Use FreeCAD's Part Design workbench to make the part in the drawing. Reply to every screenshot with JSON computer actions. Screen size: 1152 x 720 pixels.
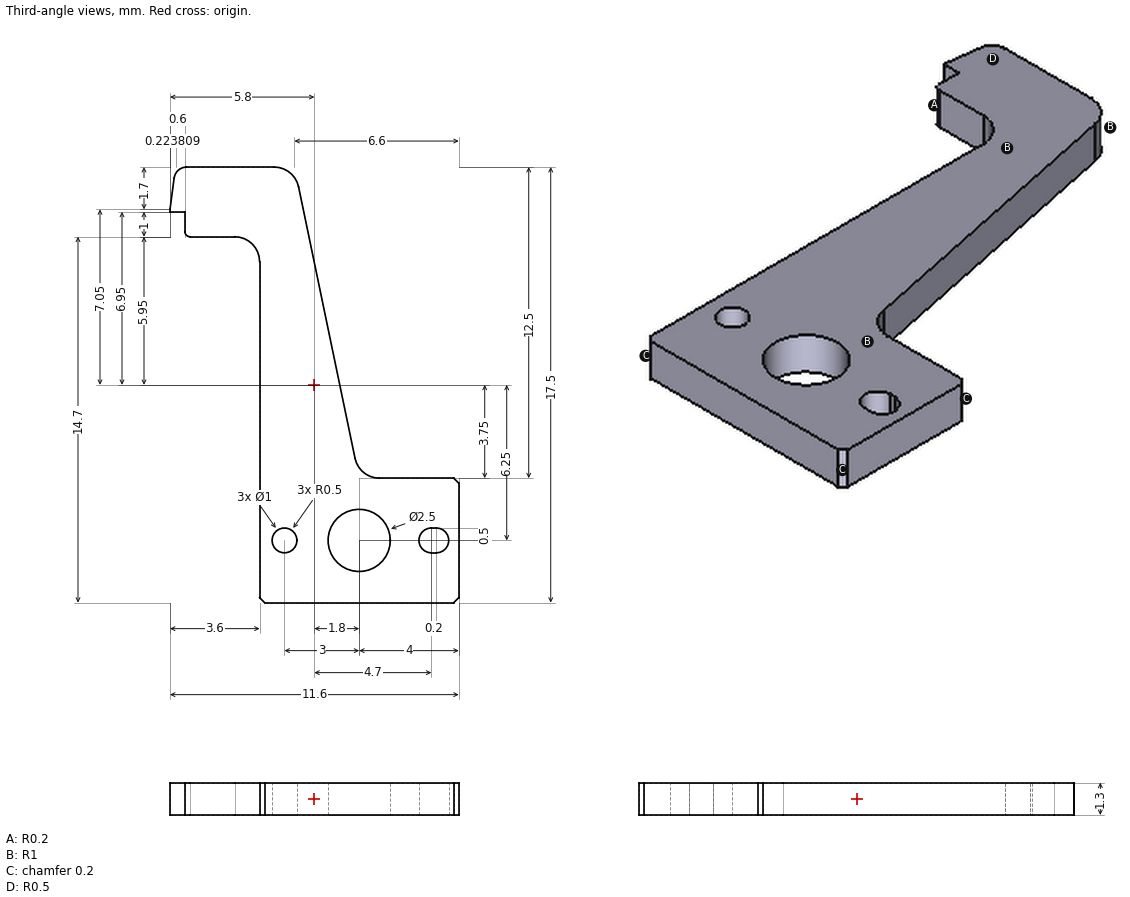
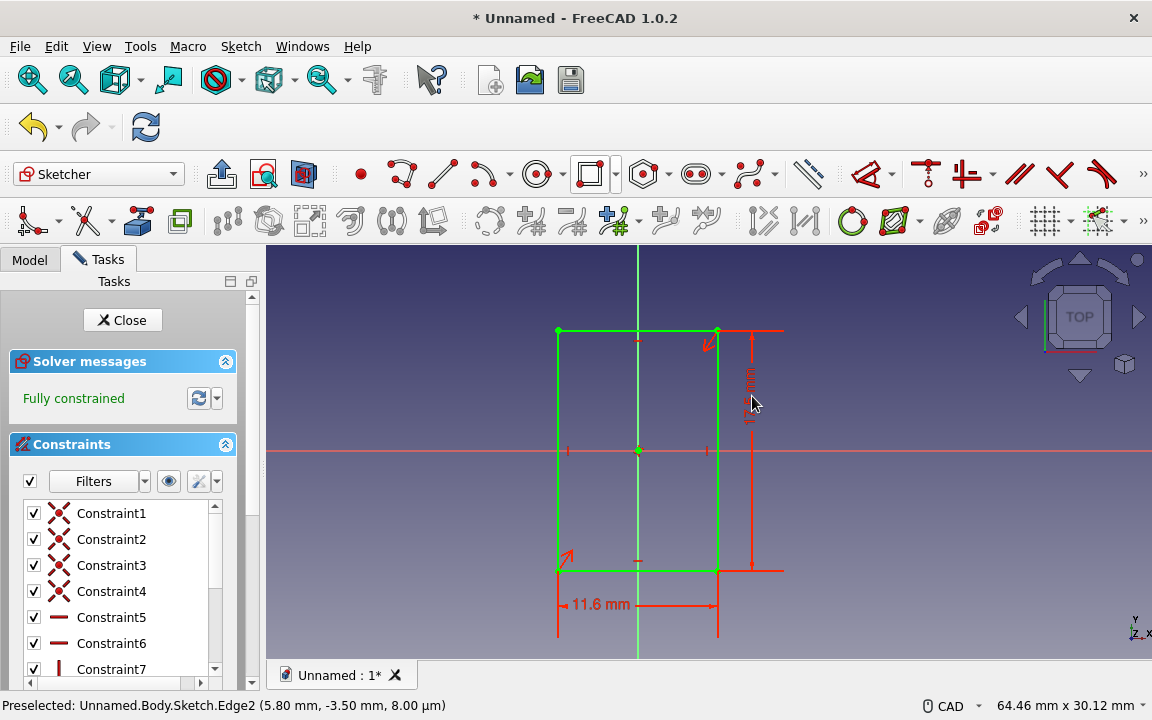
{"action": "left_click", "coordinate": [123, 320]}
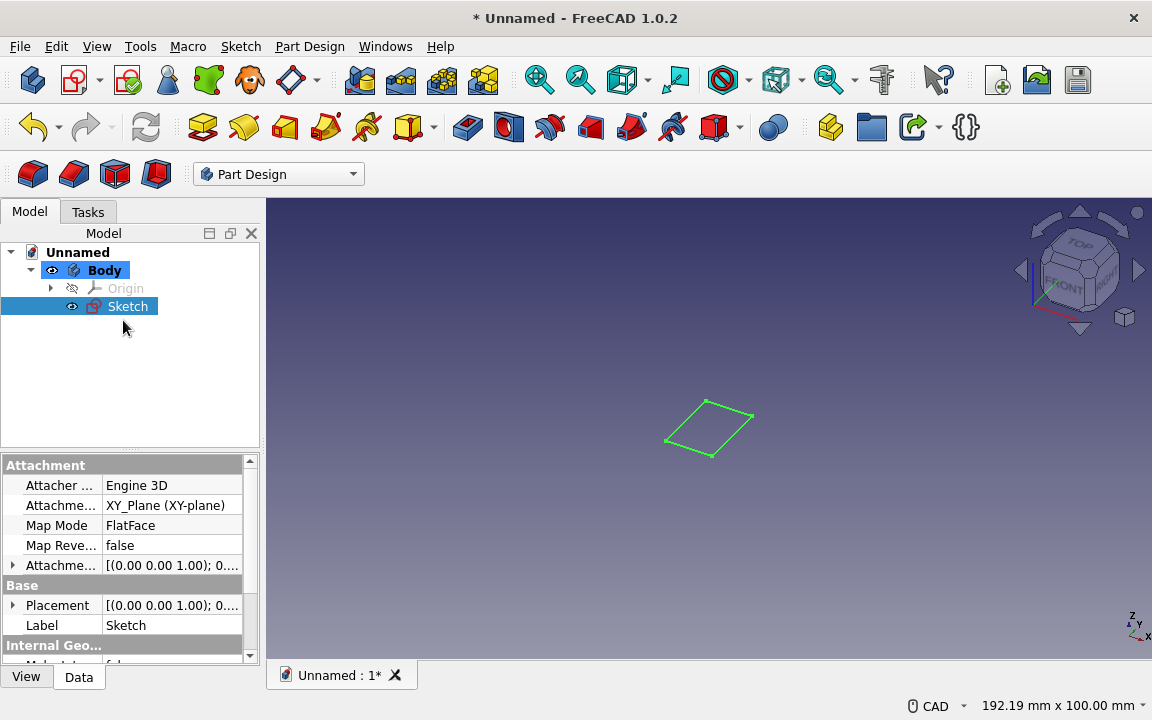
{"action": "left_click", "coordinate": [203, 128]}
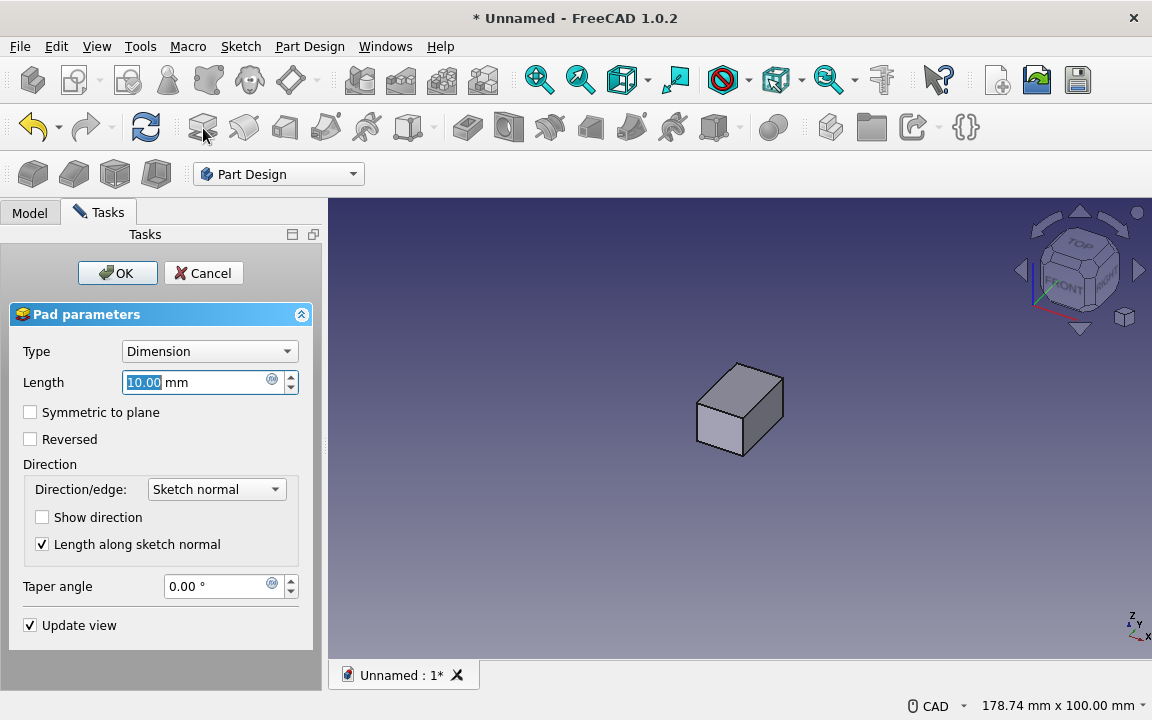
{"action": "type", "text": "1.3"}
{"action": "key", "text": "Tab"}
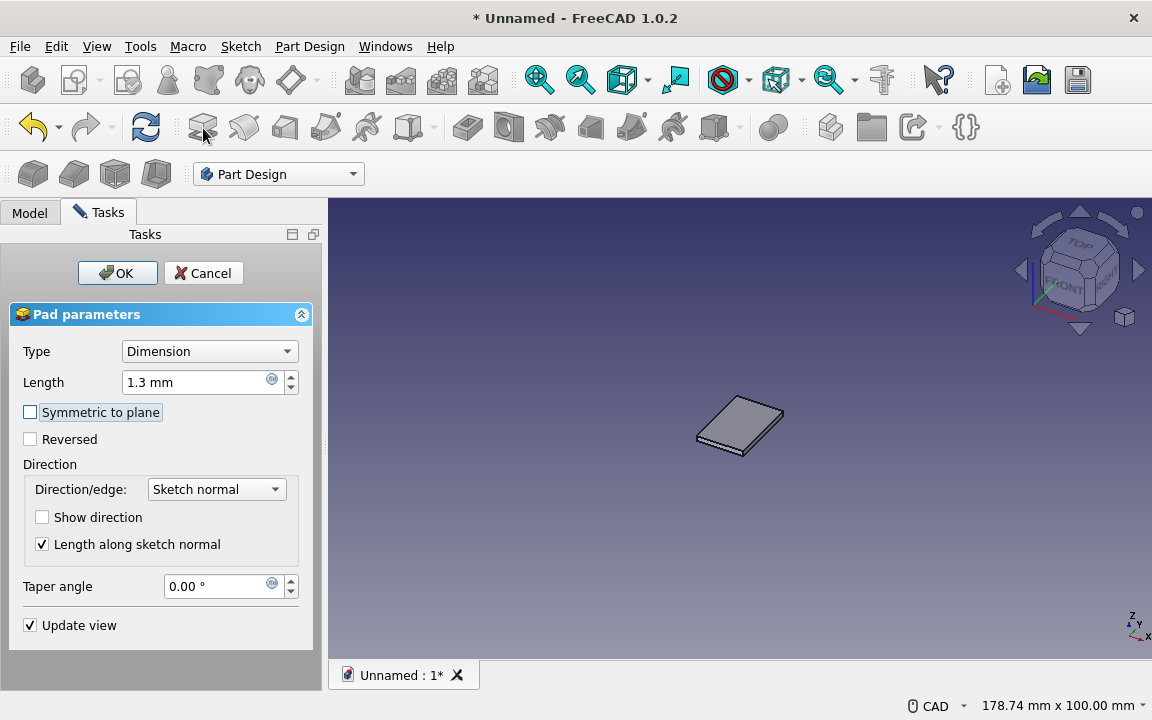
{"action": "left_click", "coordinate": [31, 412]}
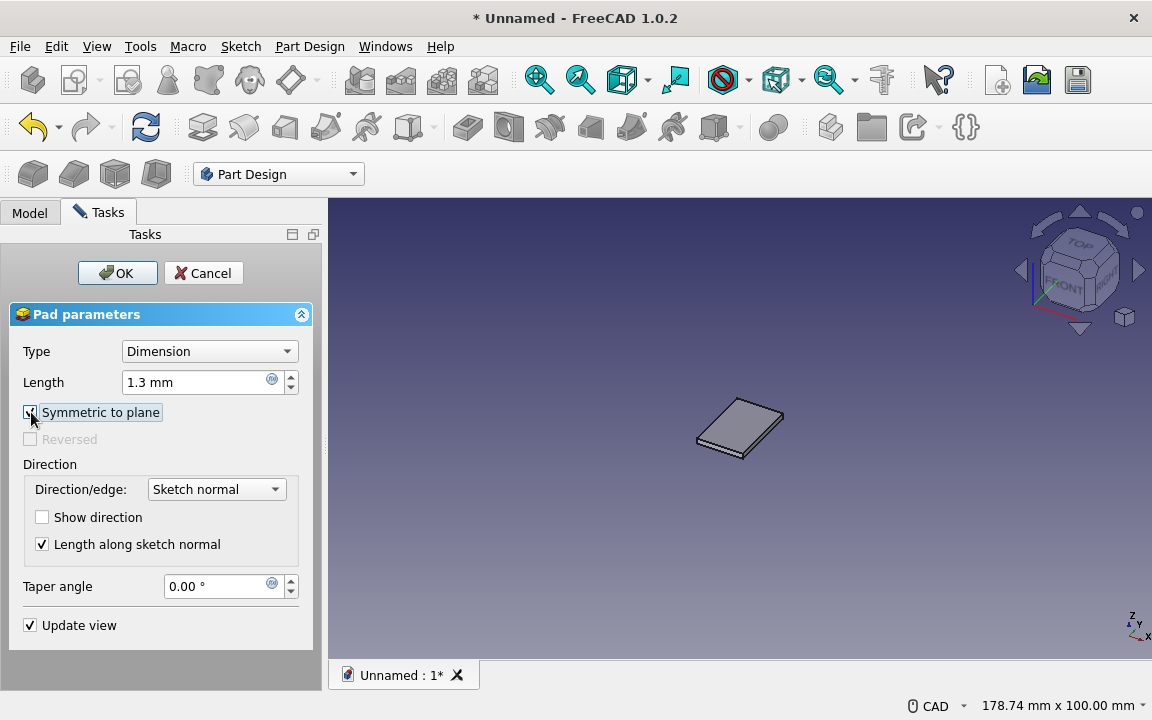
{"action": "left_click", "coordinate": [118, 273]}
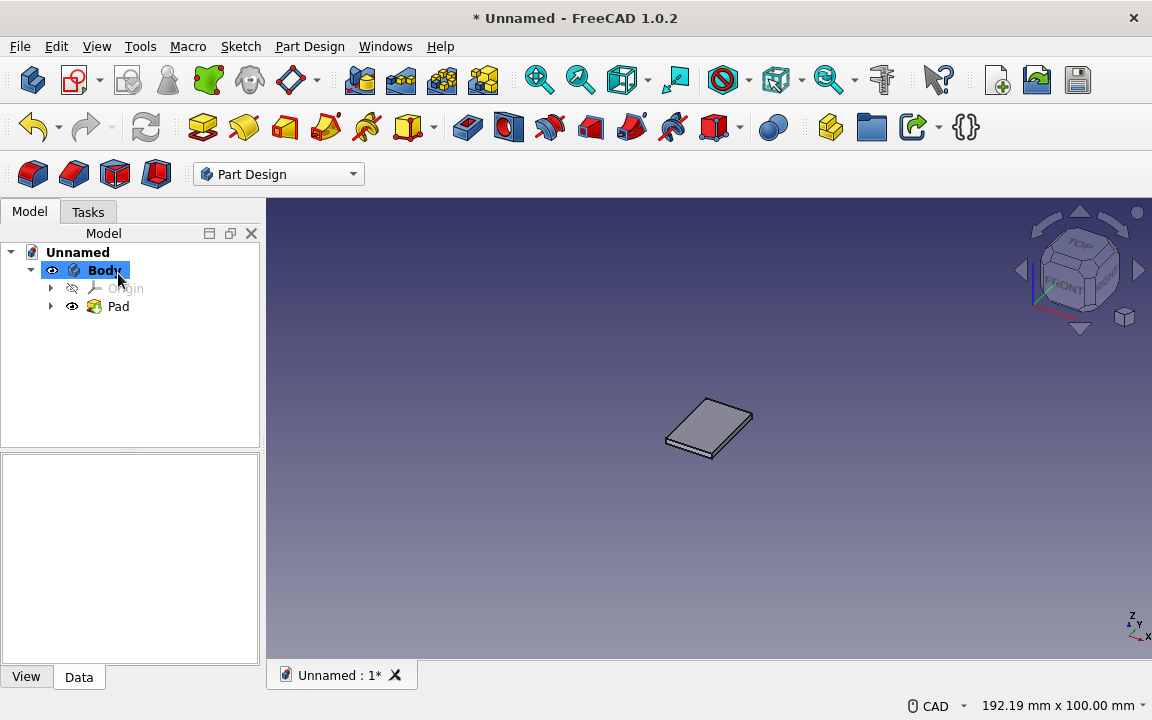
{"action": "key", "text": "v f"}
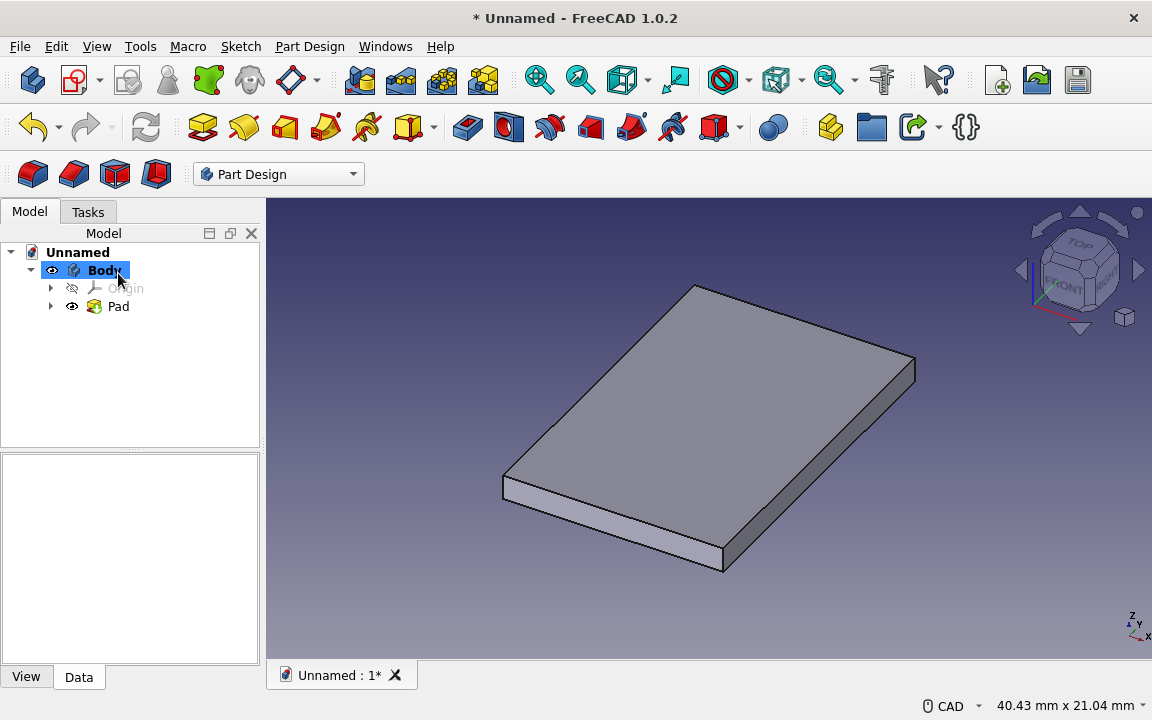
{"action": "left_click", "coordinate": [736, 389]}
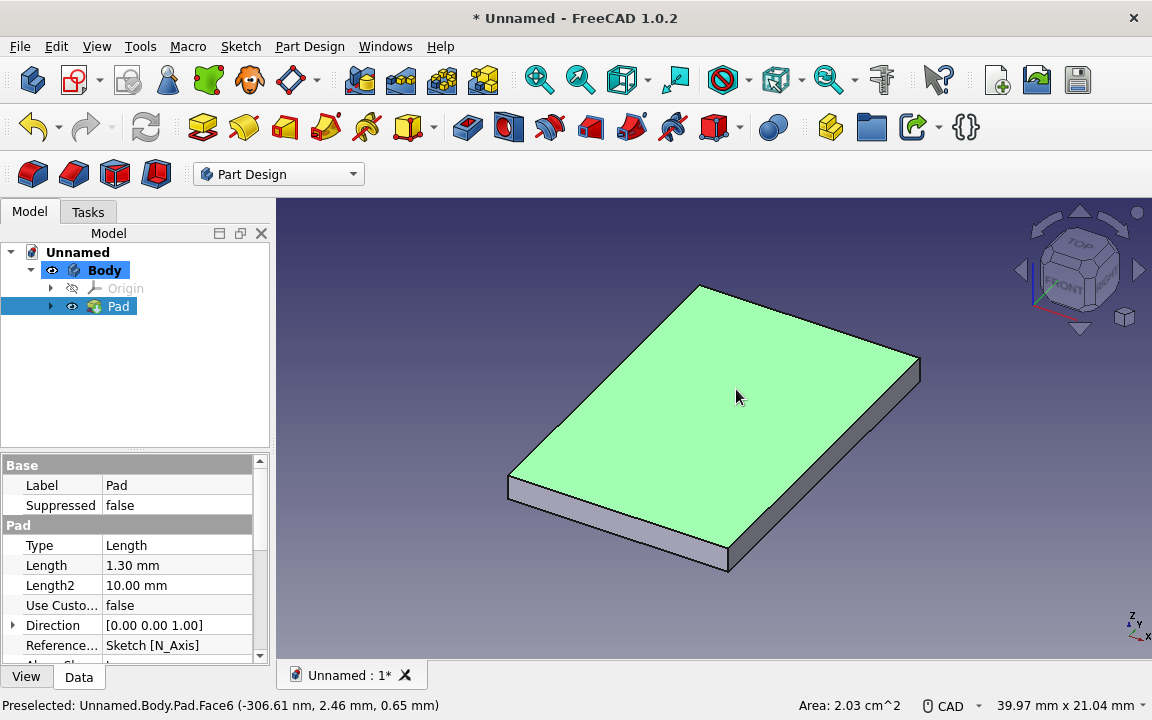
{"action": "left_click", "coordinate": [74, 80]}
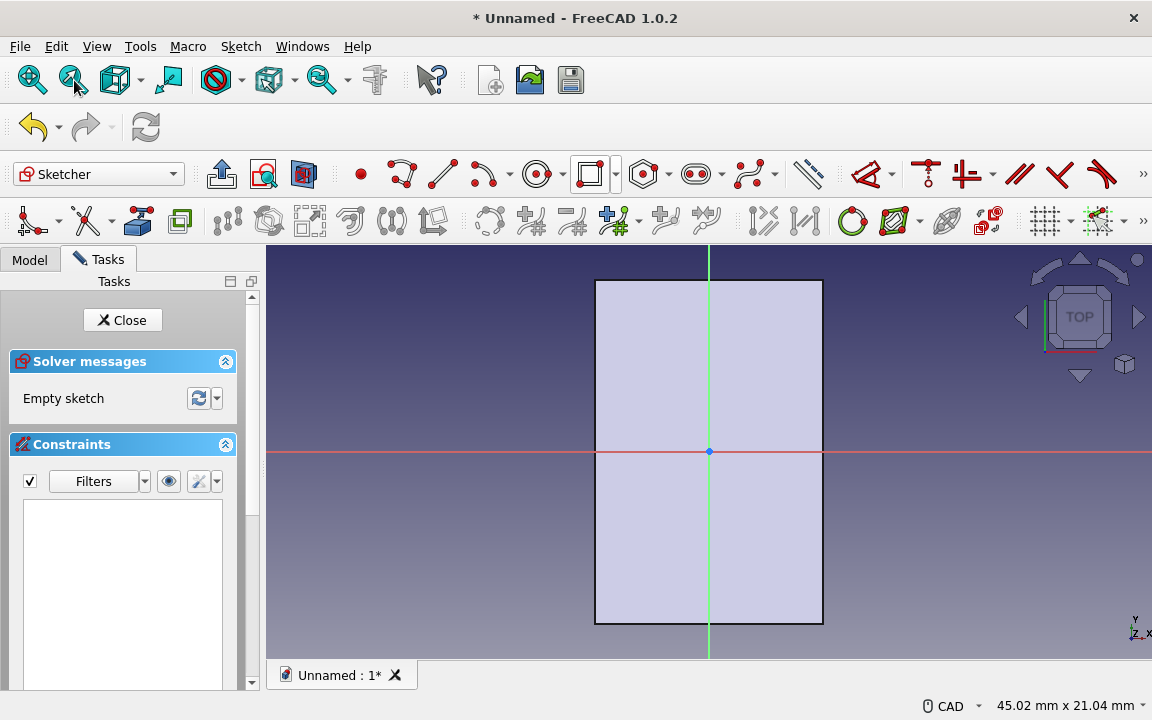
{"action": "scroll", "coordinate": [873, 616], "scroll_direction": "up", "scroll_amount": 3}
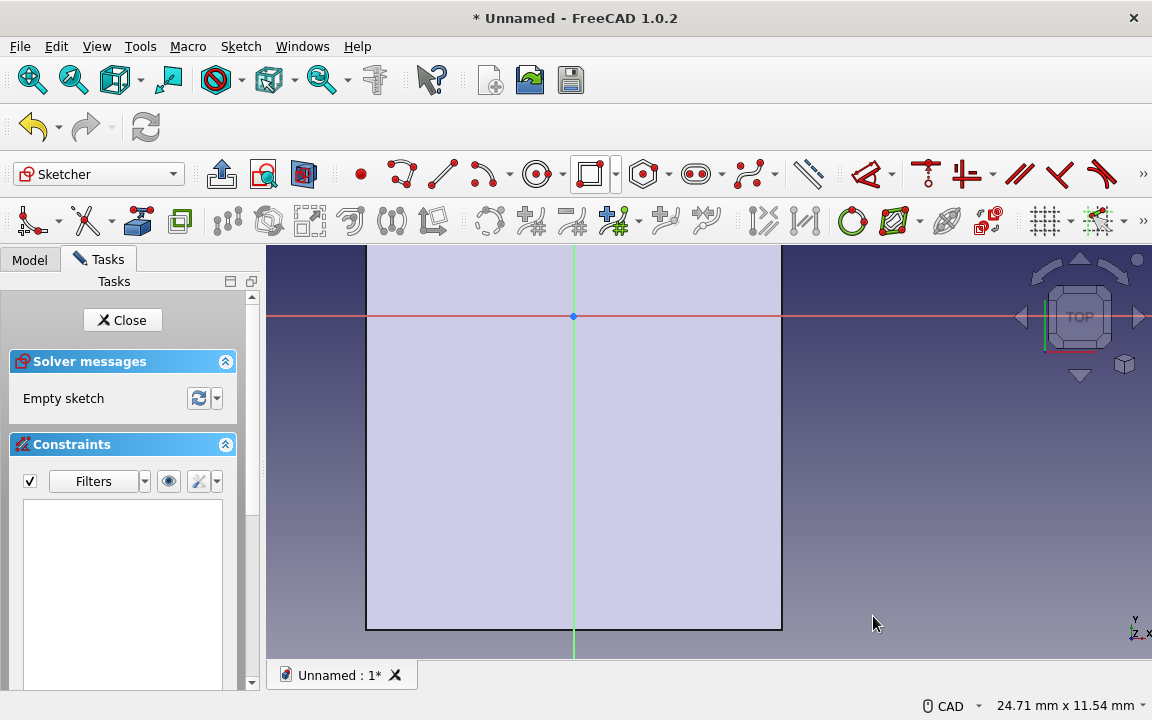
{"action": "key", "text": "g s"}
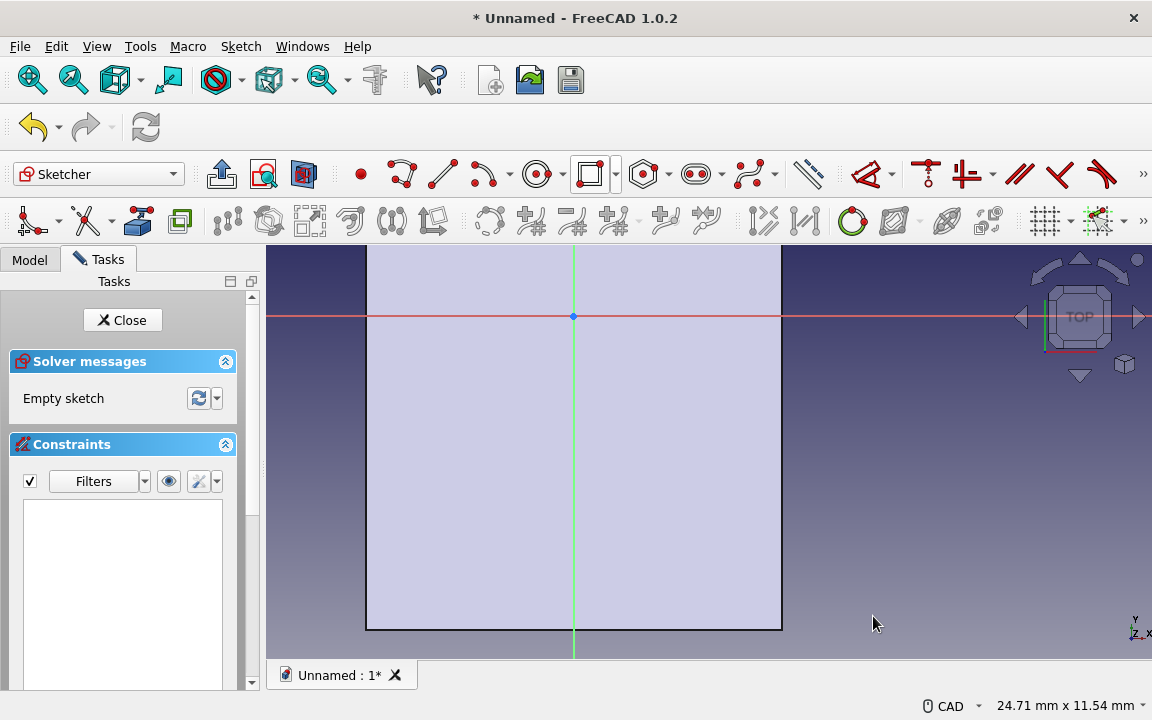
{"action": "scroll", "coordinate": [742, 541], "scroll_direction": "up", "scroll_amount": 2}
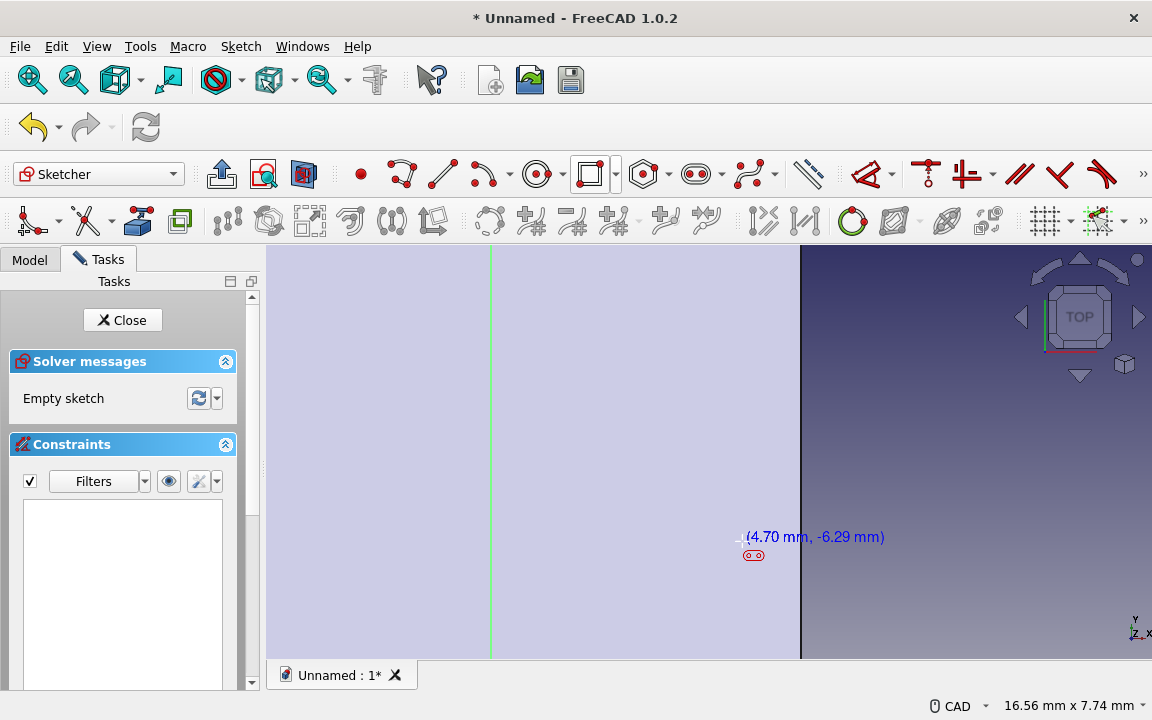
{"action": "left_click", "coordinate": [742, 540]}